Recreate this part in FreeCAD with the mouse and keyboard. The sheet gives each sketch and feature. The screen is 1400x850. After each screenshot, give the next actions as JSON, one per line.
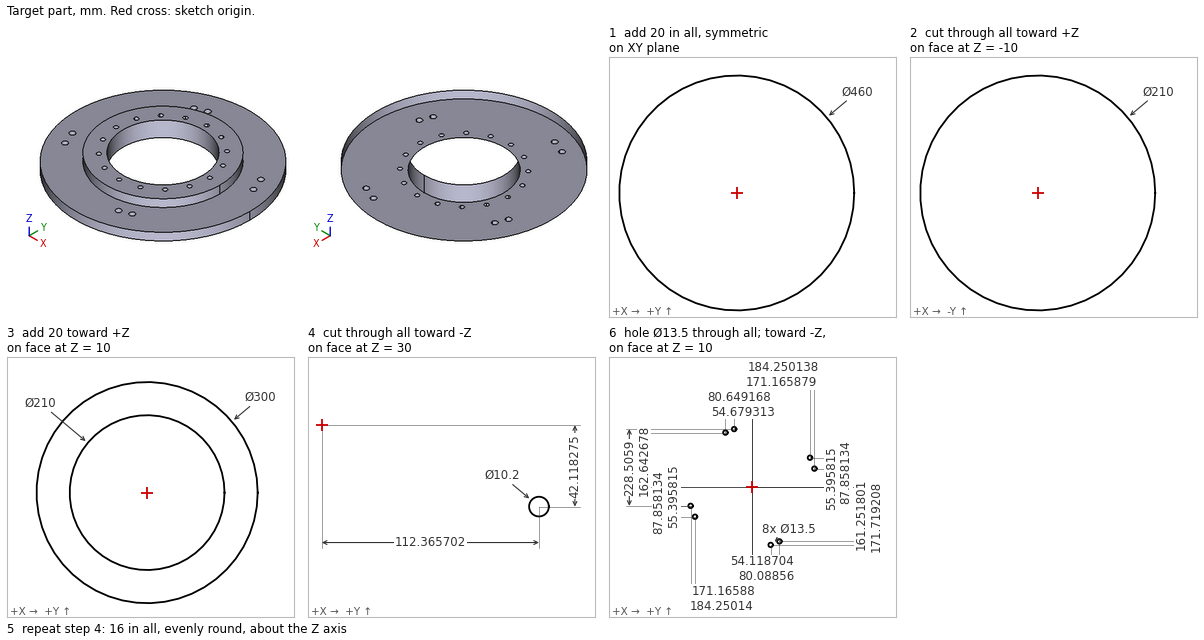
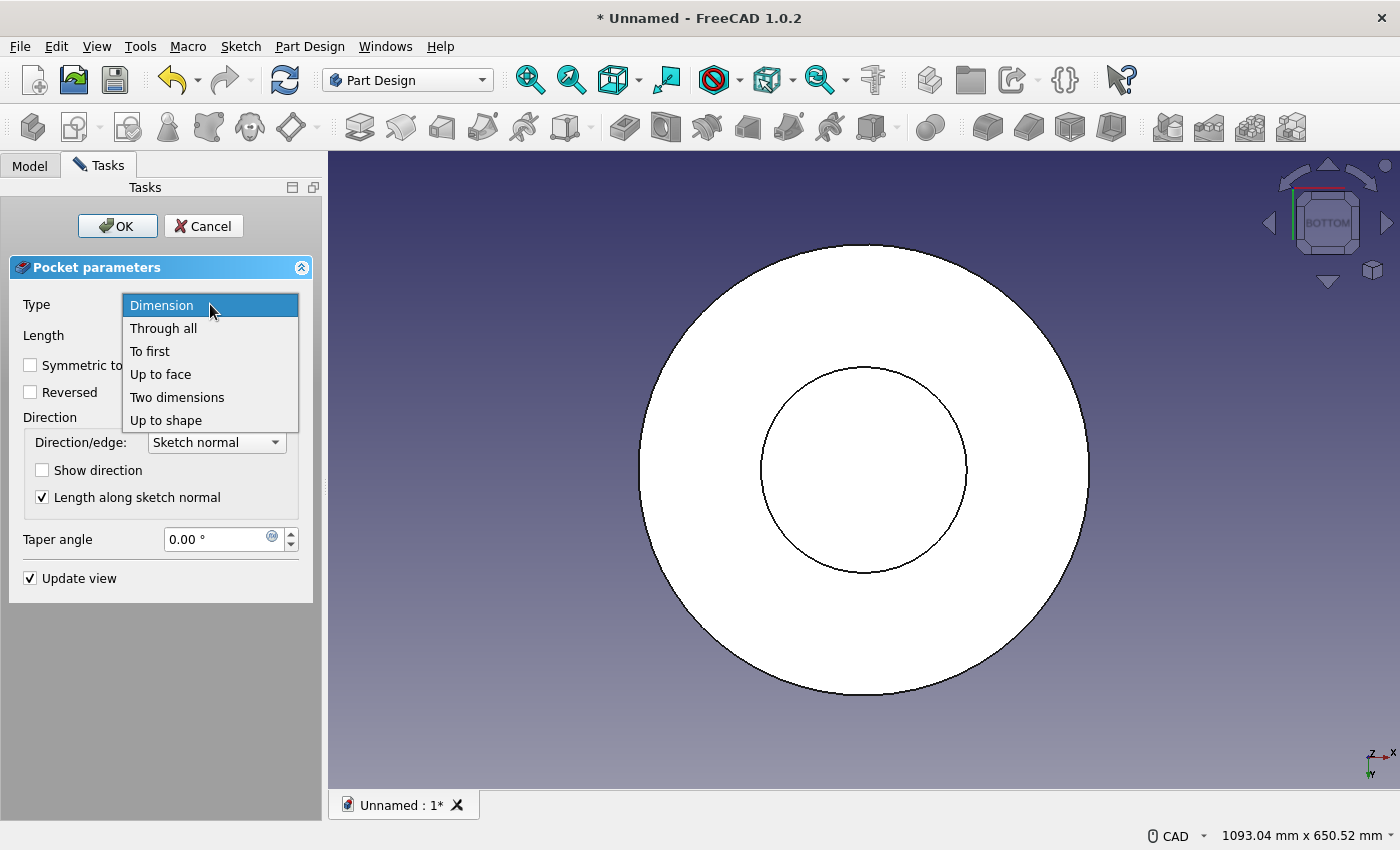
{"action": "left_click", "coordinate": [208, 328]}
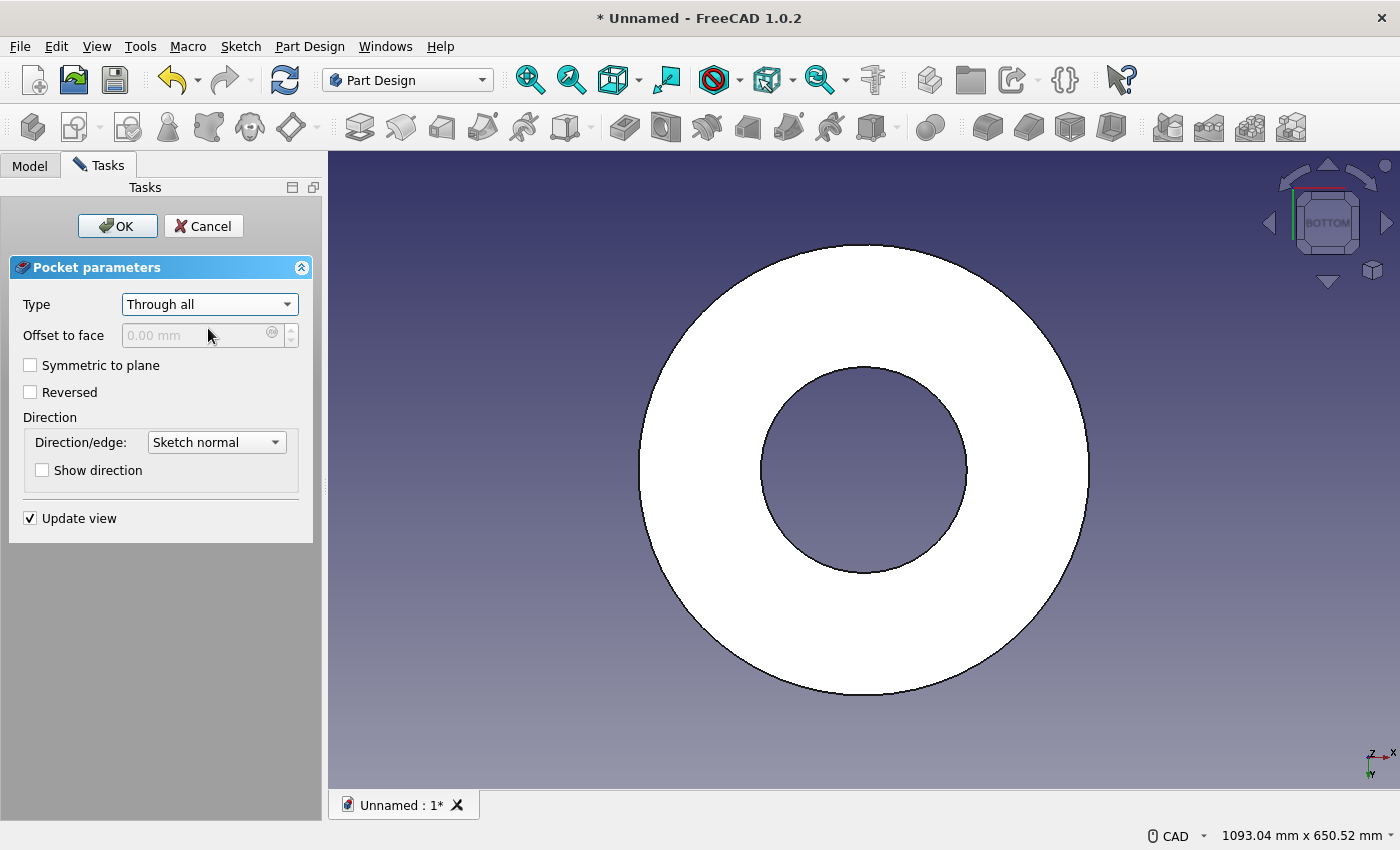
{"action": "left_click", "coordinate": [118, 226]}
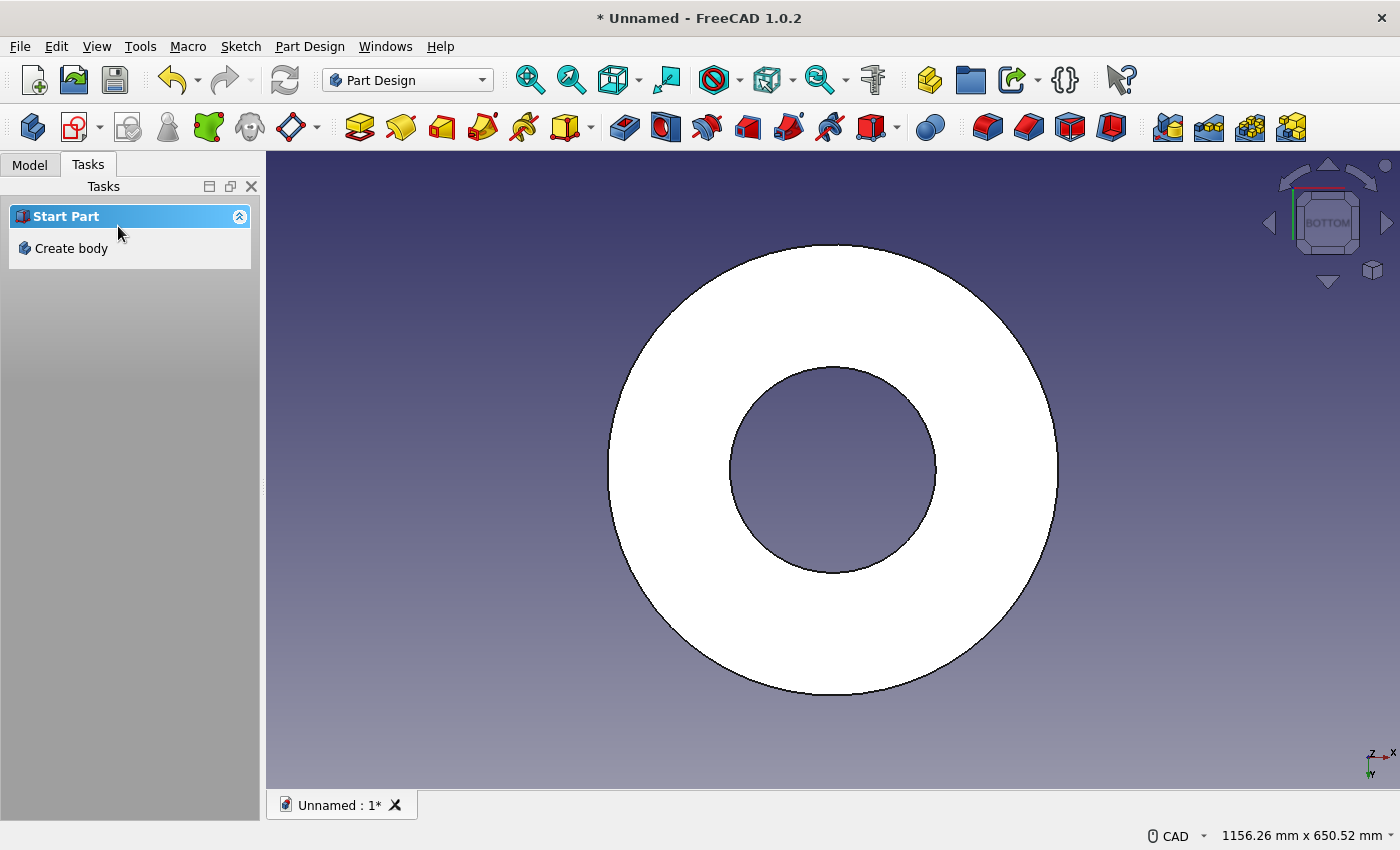
{"action": "key", "text": "0"}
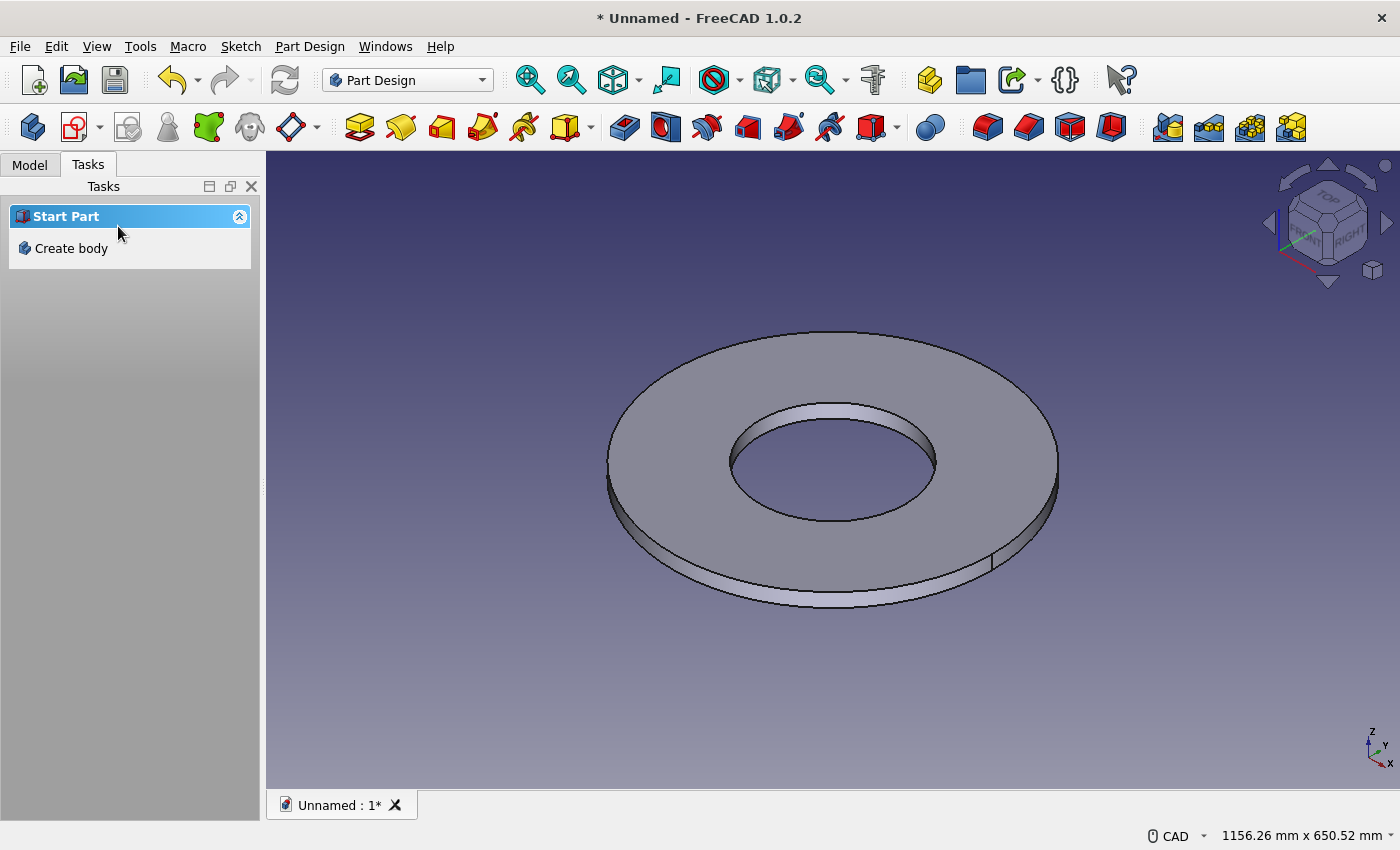
{"action": "left_click", "coordinate": [651, 461]}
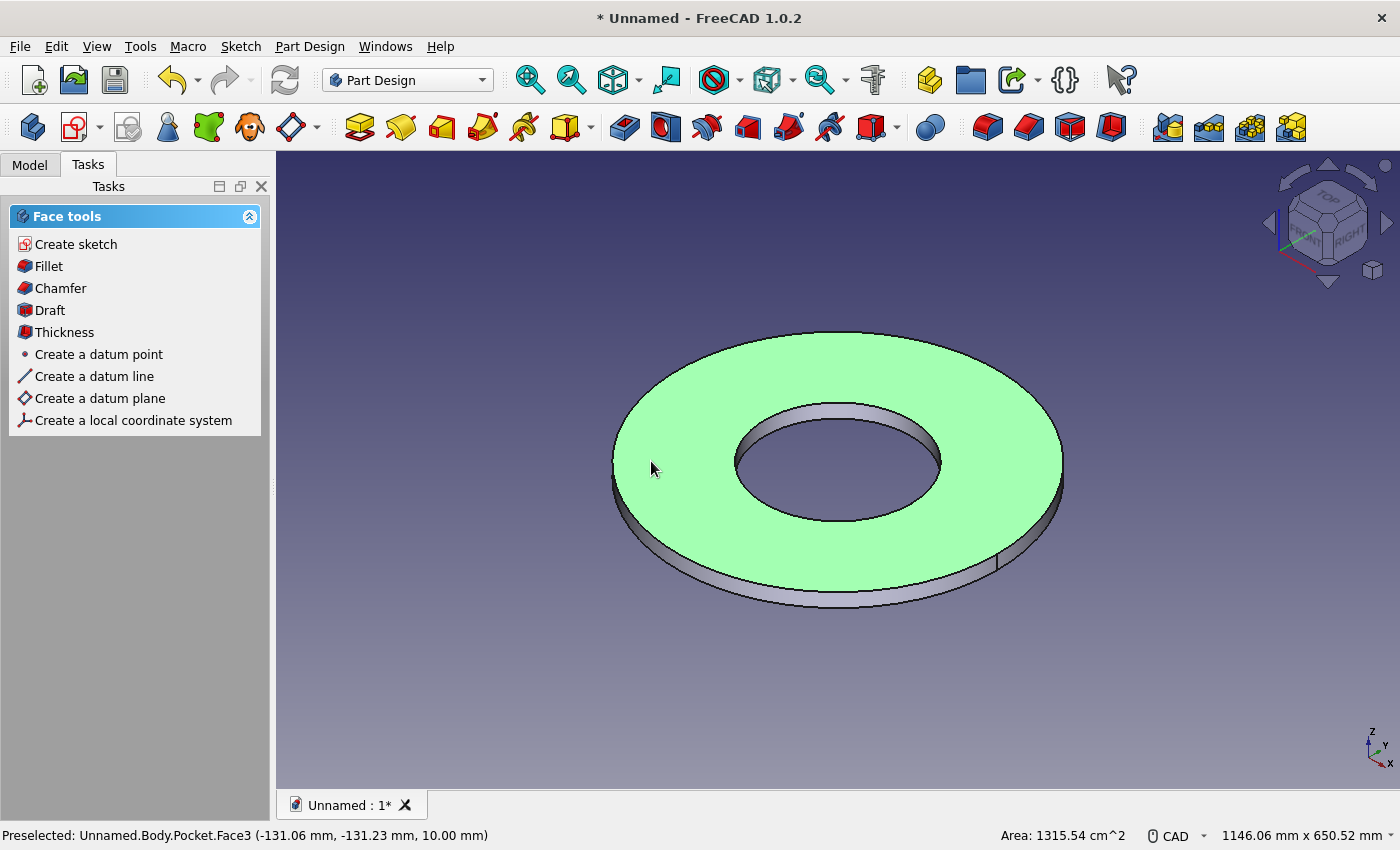
{"action": "left_click", "coordinate": [74, 128]}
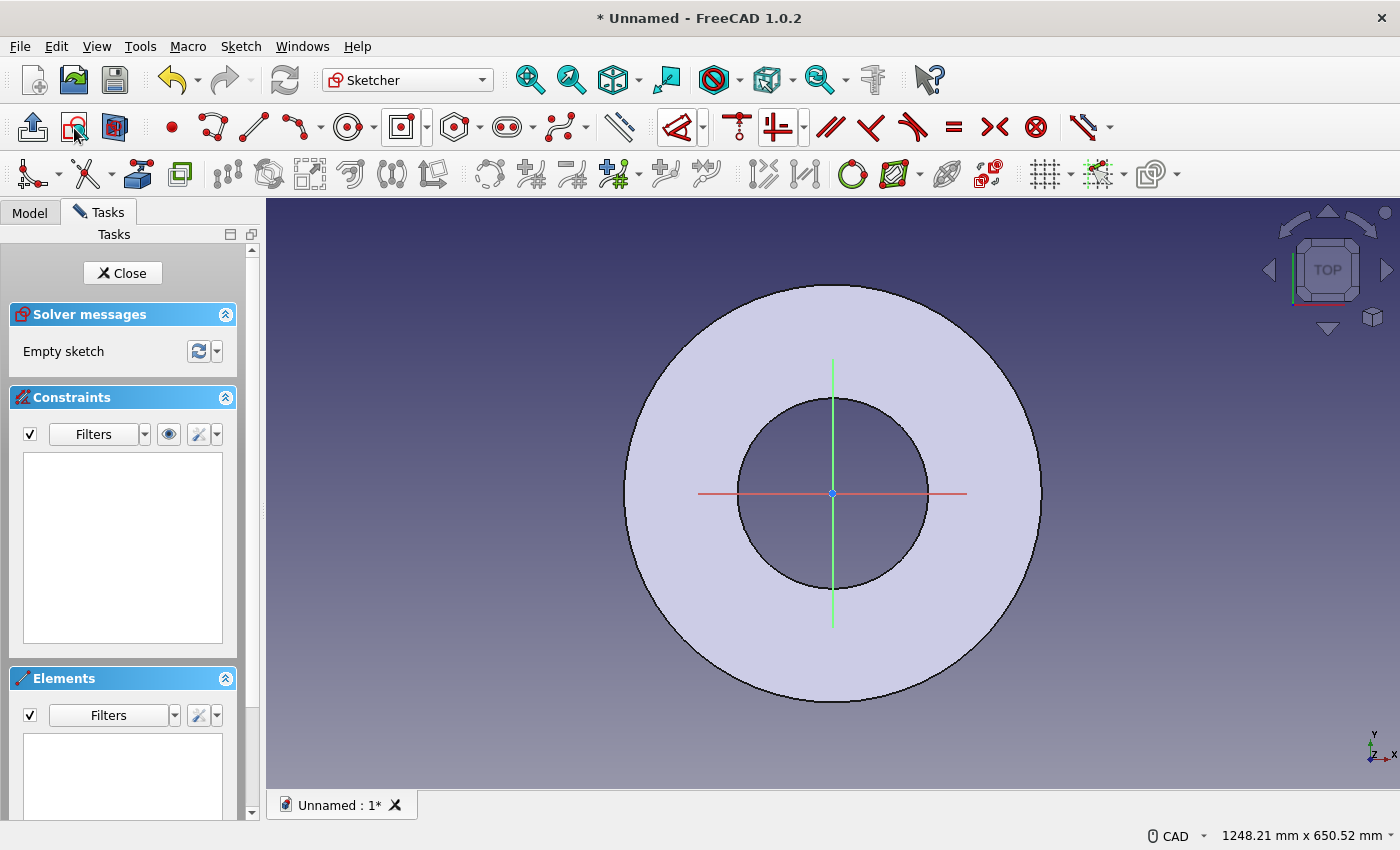
{"action": "scroll", "coordinate": [972, 493], "scroll_direction": "up", "scroll_amount": 2}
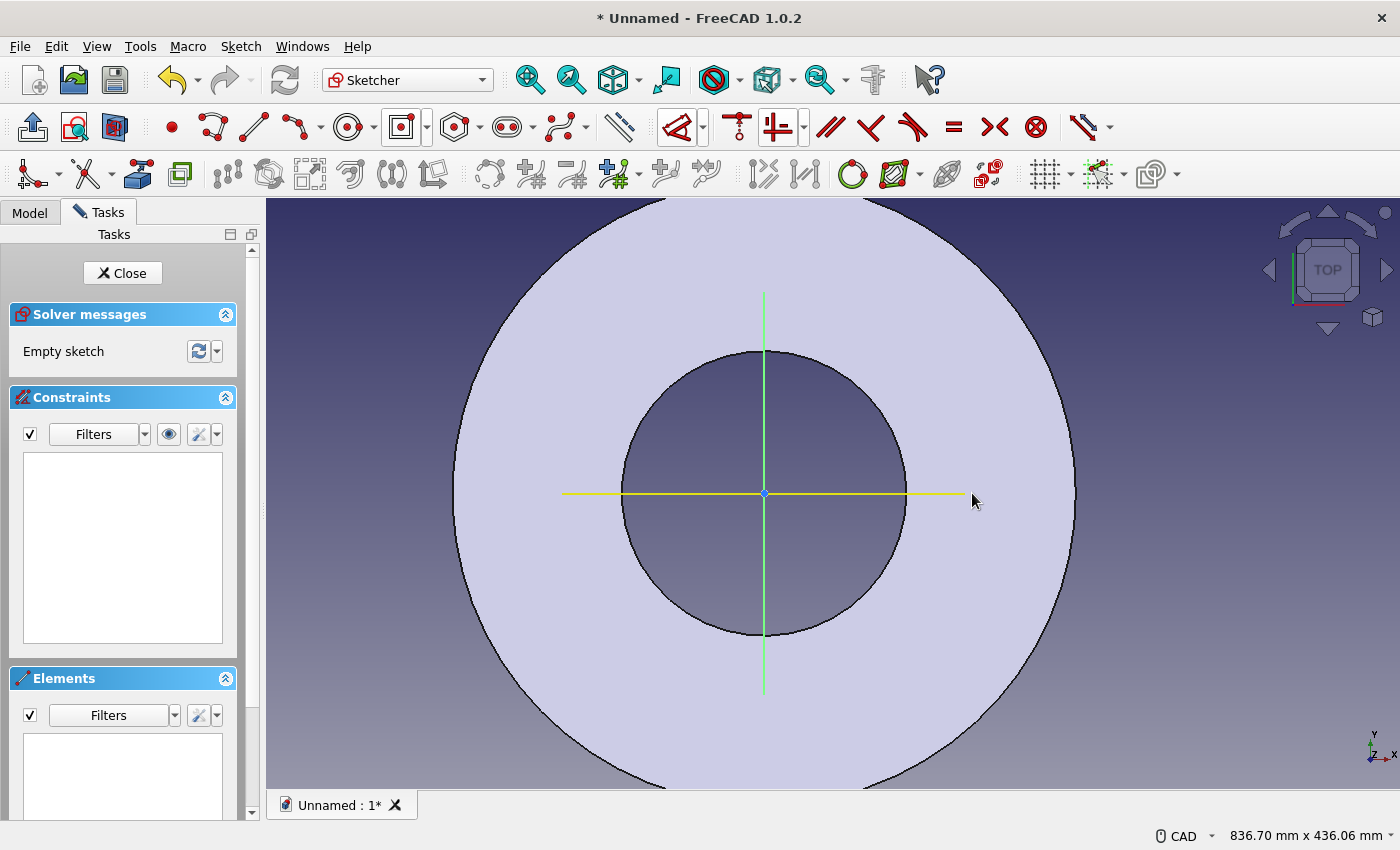
{"action": "key", "text": "g c"}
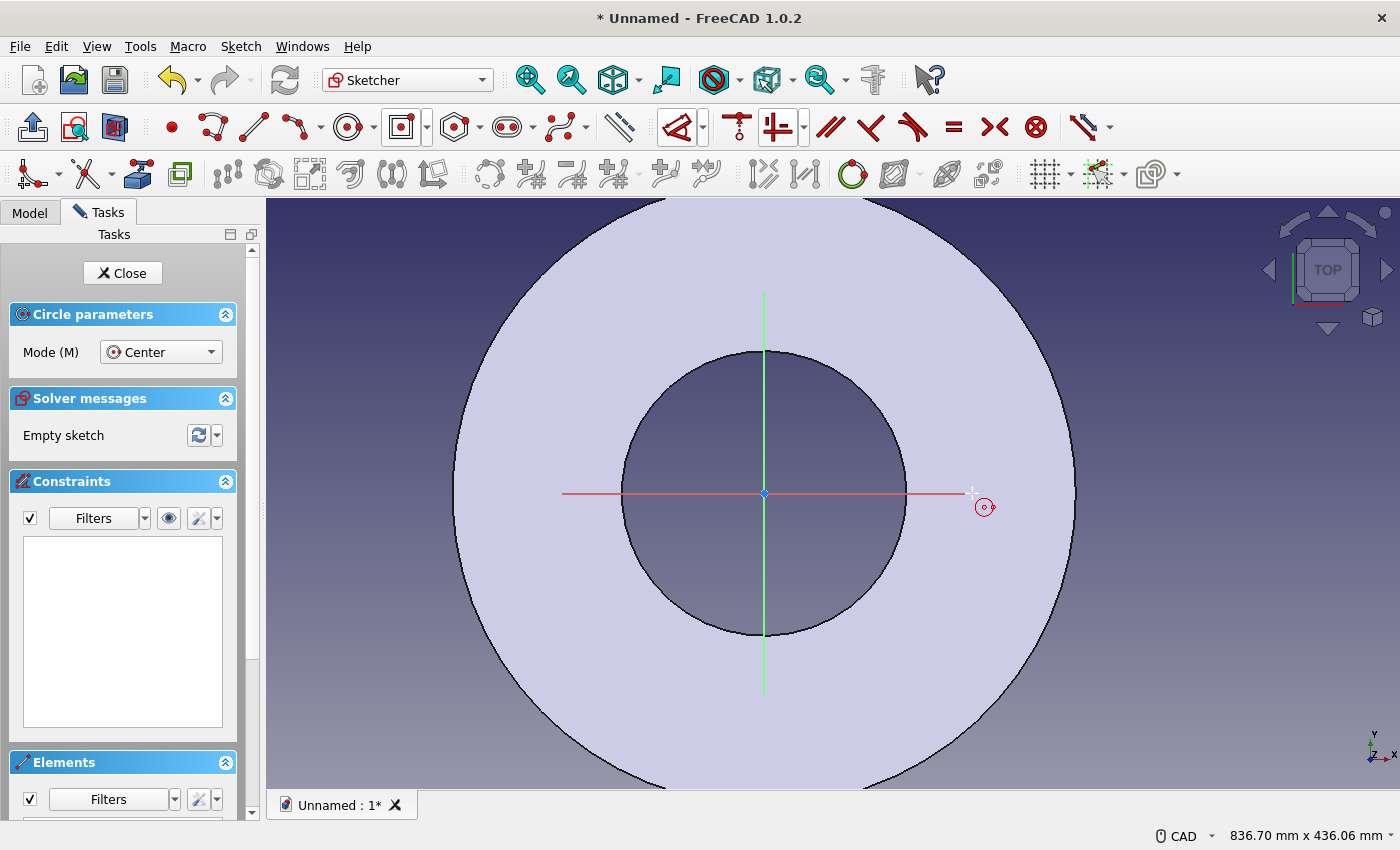
{"action": "left_click", "coordinate": [764, 493]}
{"action": "mouse_move", "coordinate": [908, 350]}